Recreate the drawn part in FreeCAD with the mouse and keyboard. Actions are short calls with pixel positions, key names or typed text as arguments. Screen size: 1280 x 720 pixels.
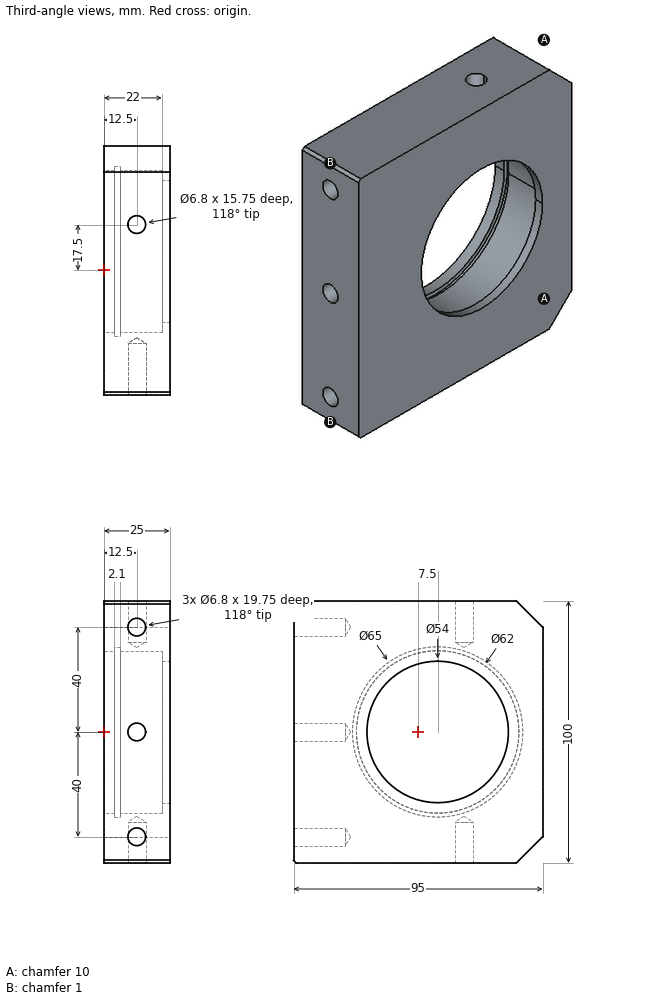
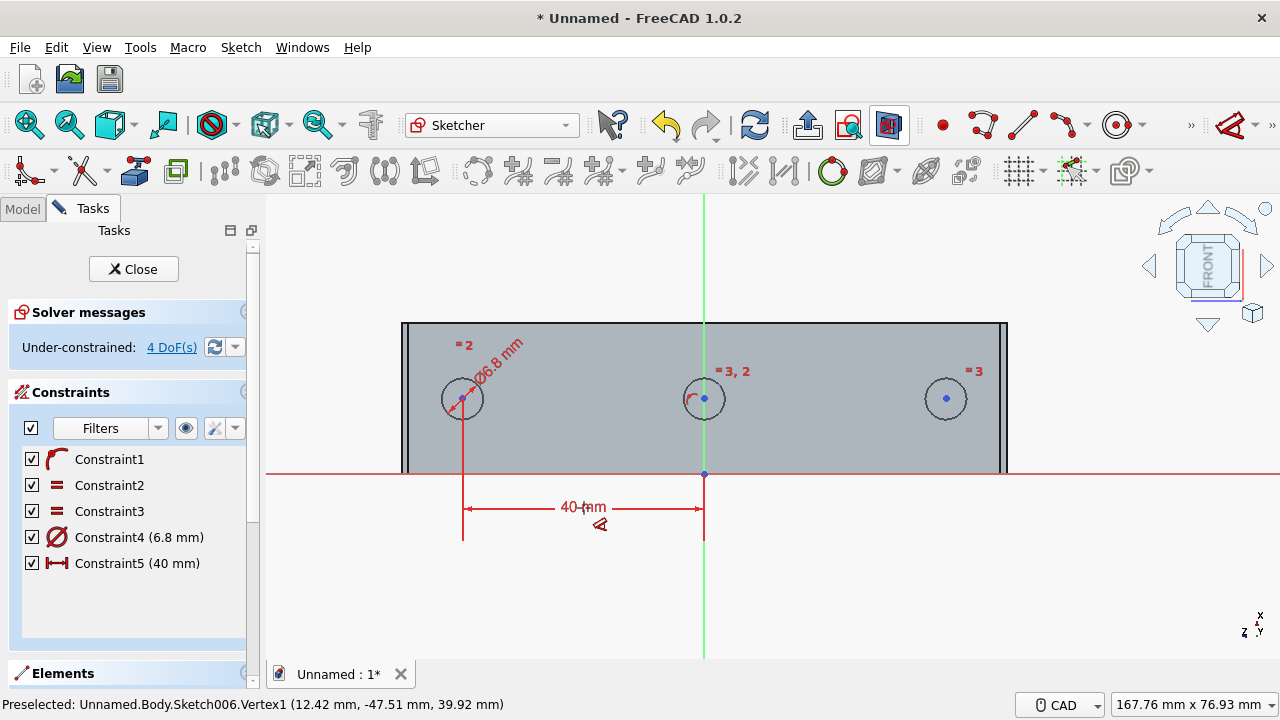
click(946, 399)
click(825, 508)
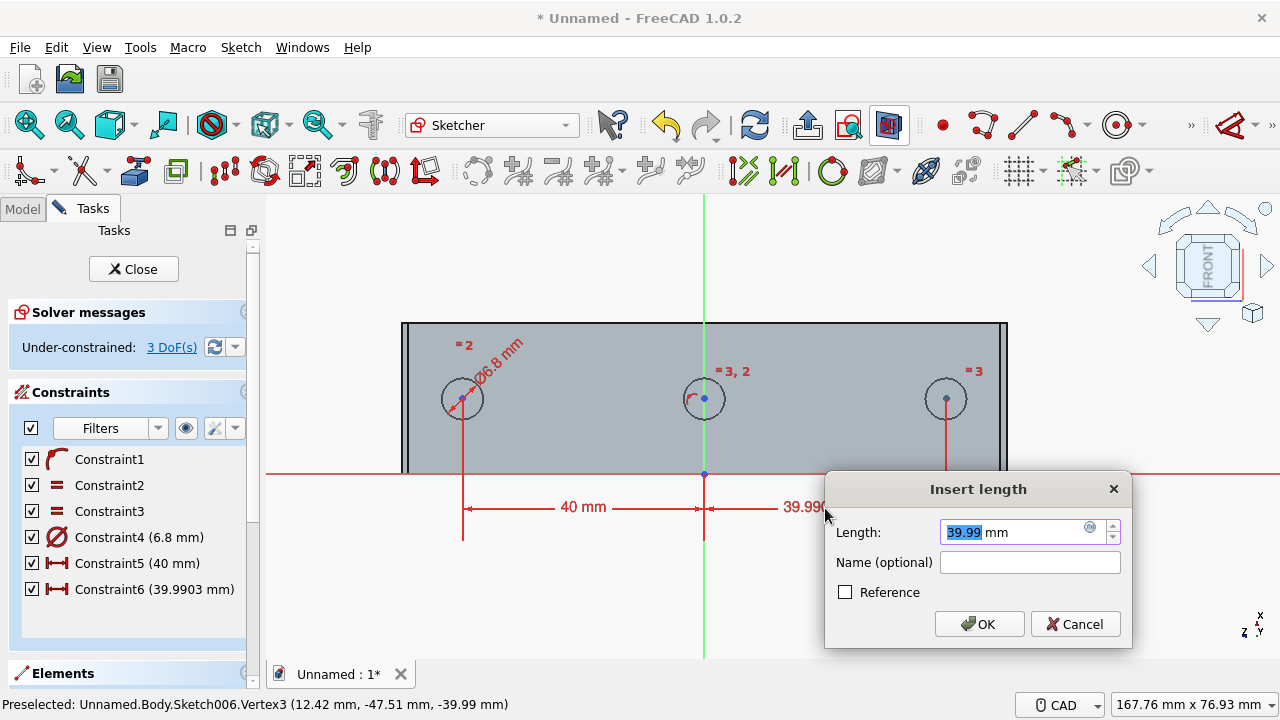
text(40)
key(Return)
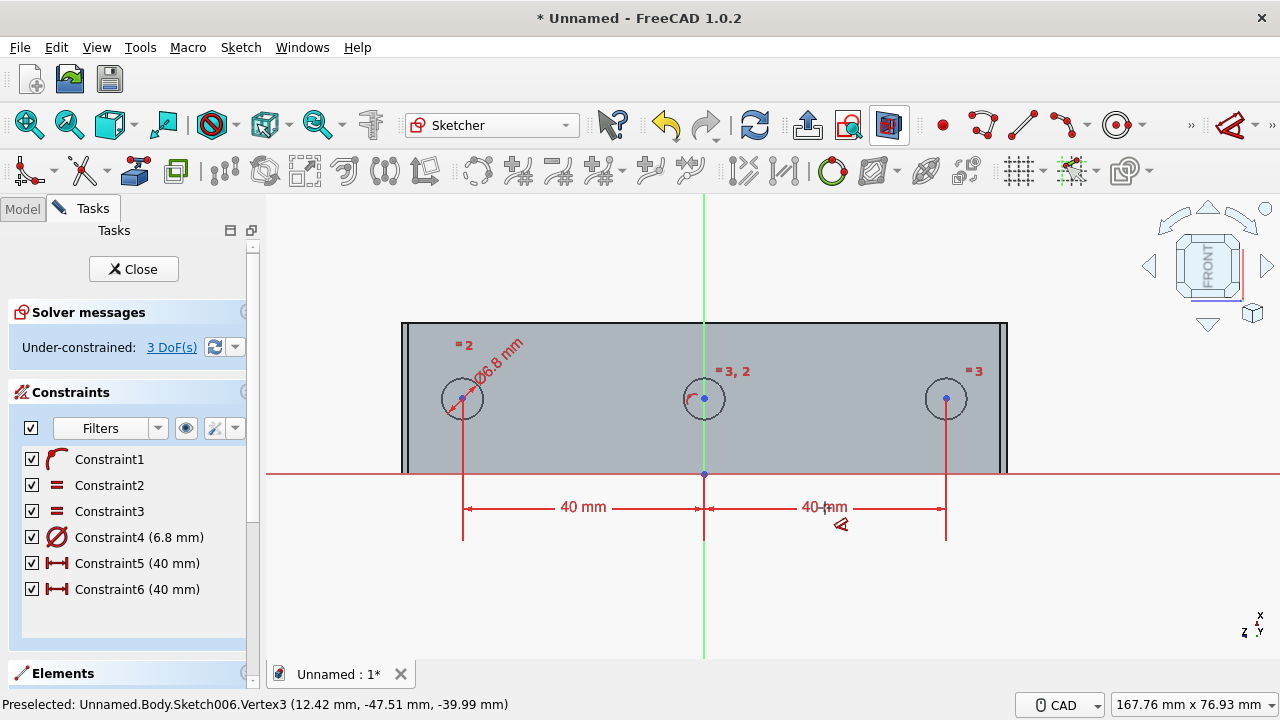
click(463, 399)
click(429, 437)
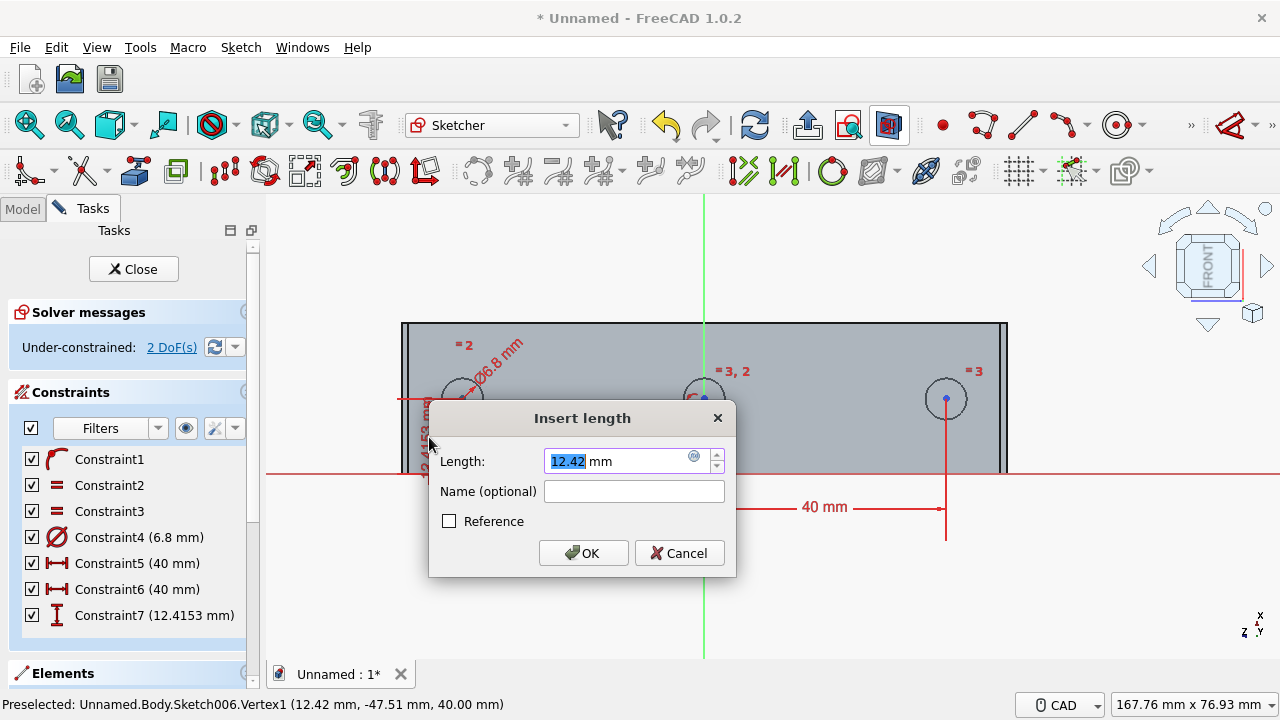
text(12.5)
key(Return)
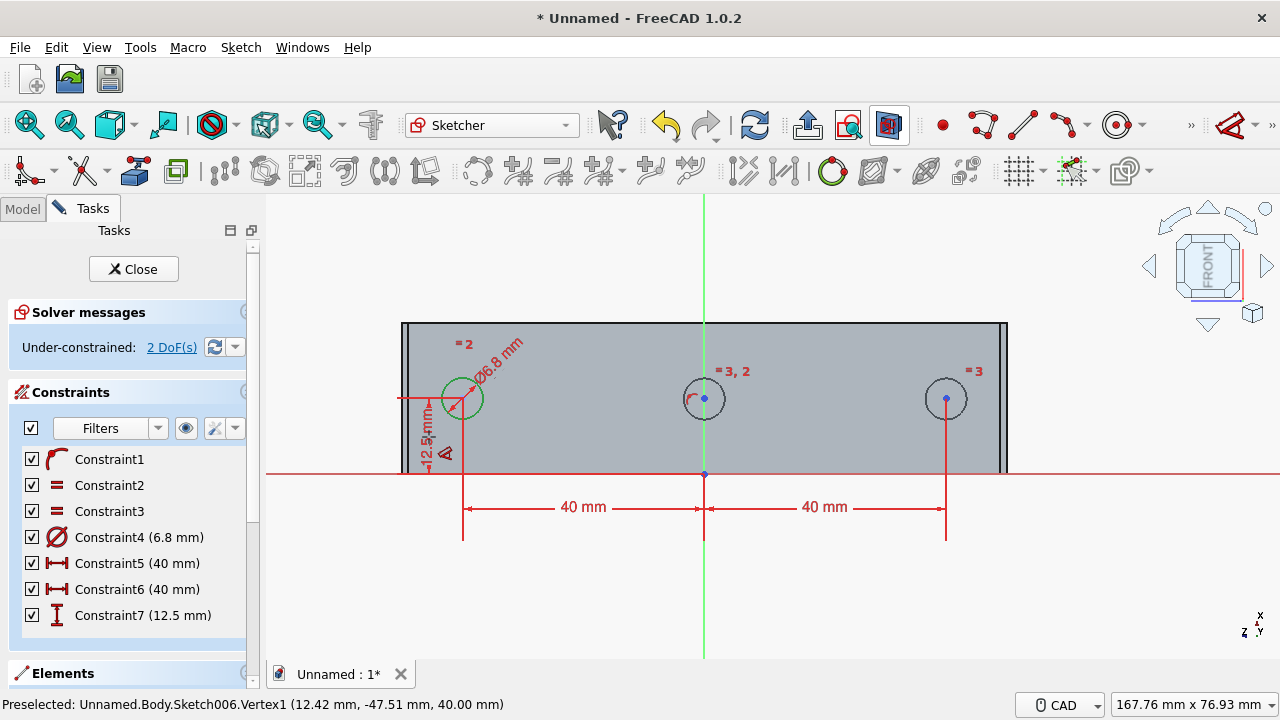
click(704, 399)
click(738, 437)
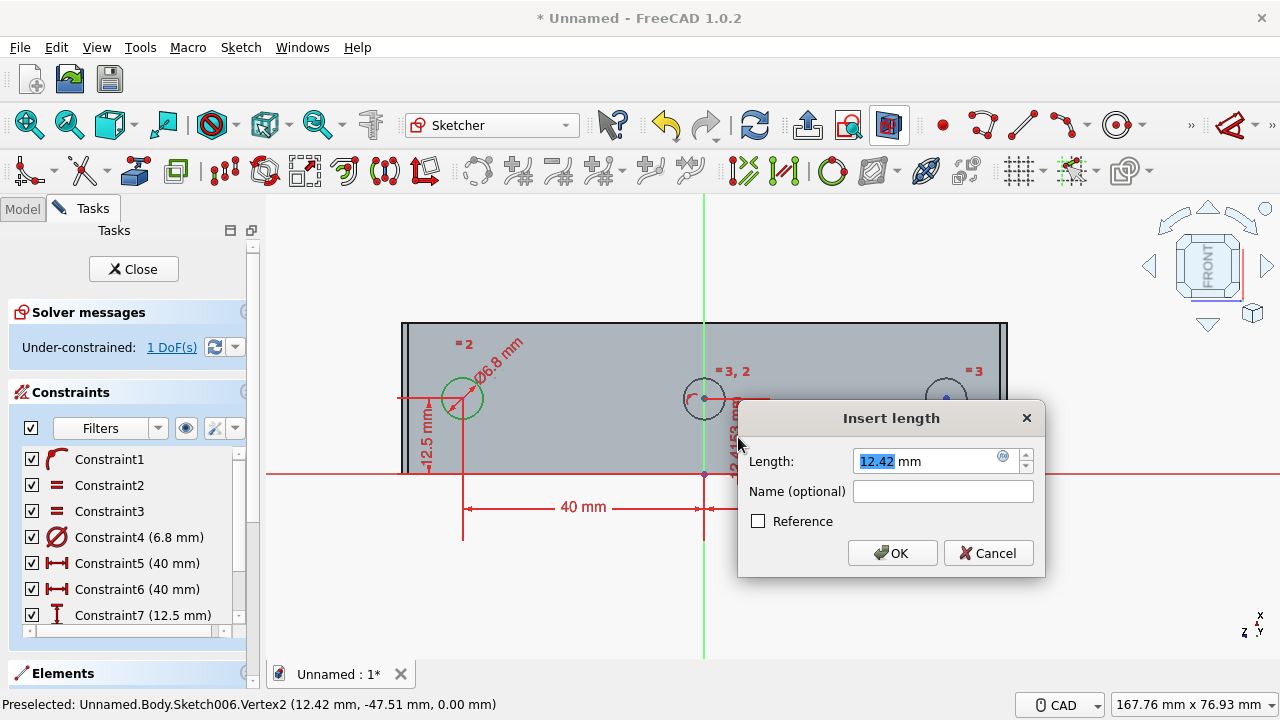
text(12.5)
key(Return)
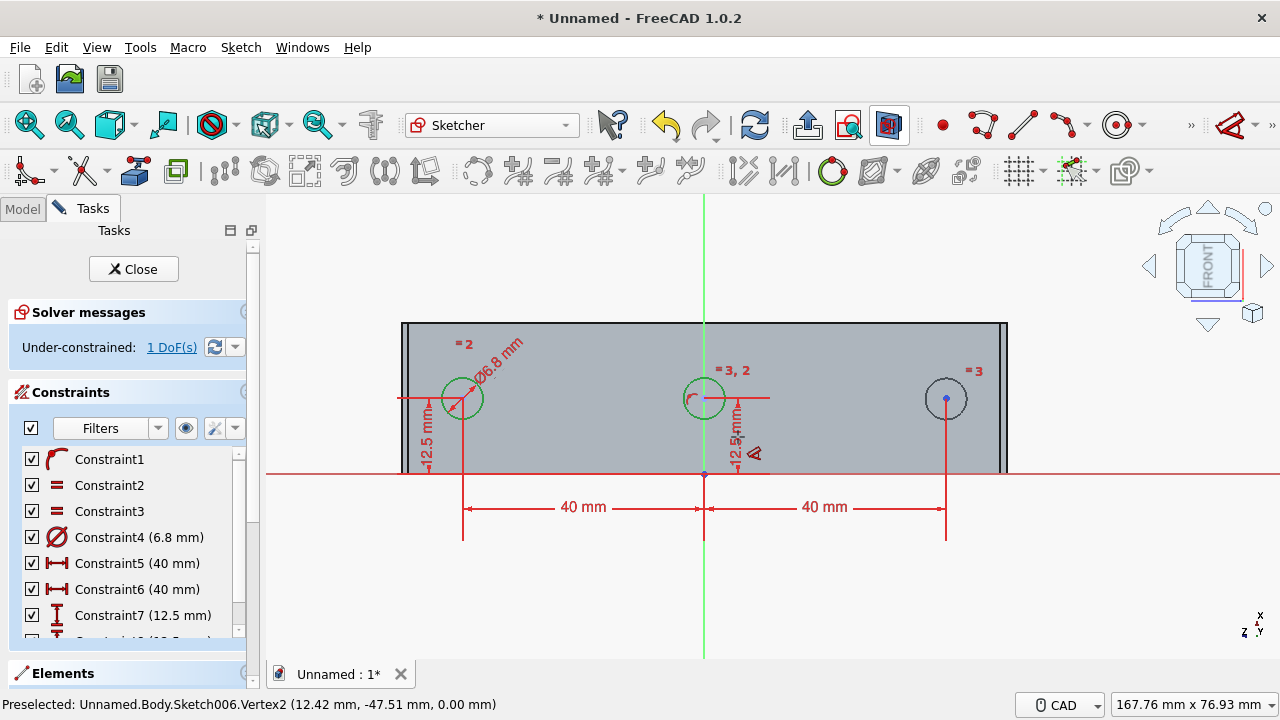
click(946, 399)
click(980, 437)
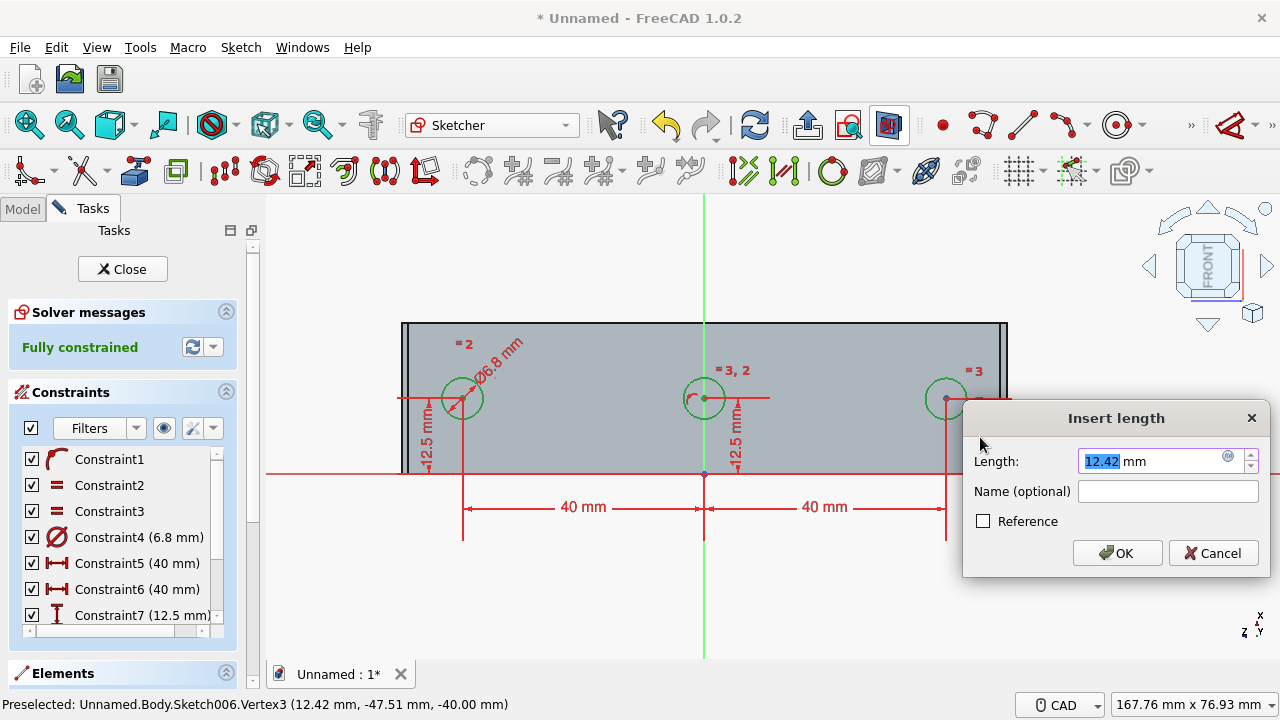
text(12.5)
key(Return)
key(Escape)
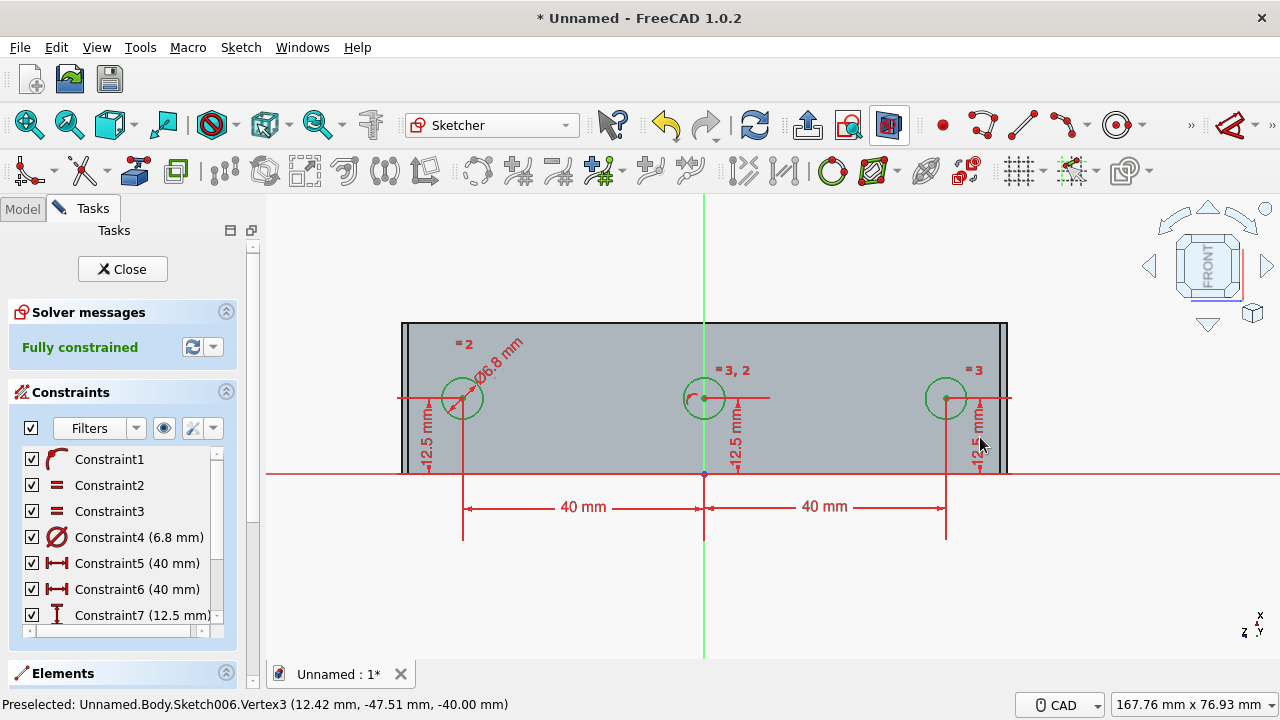
click(123, 269)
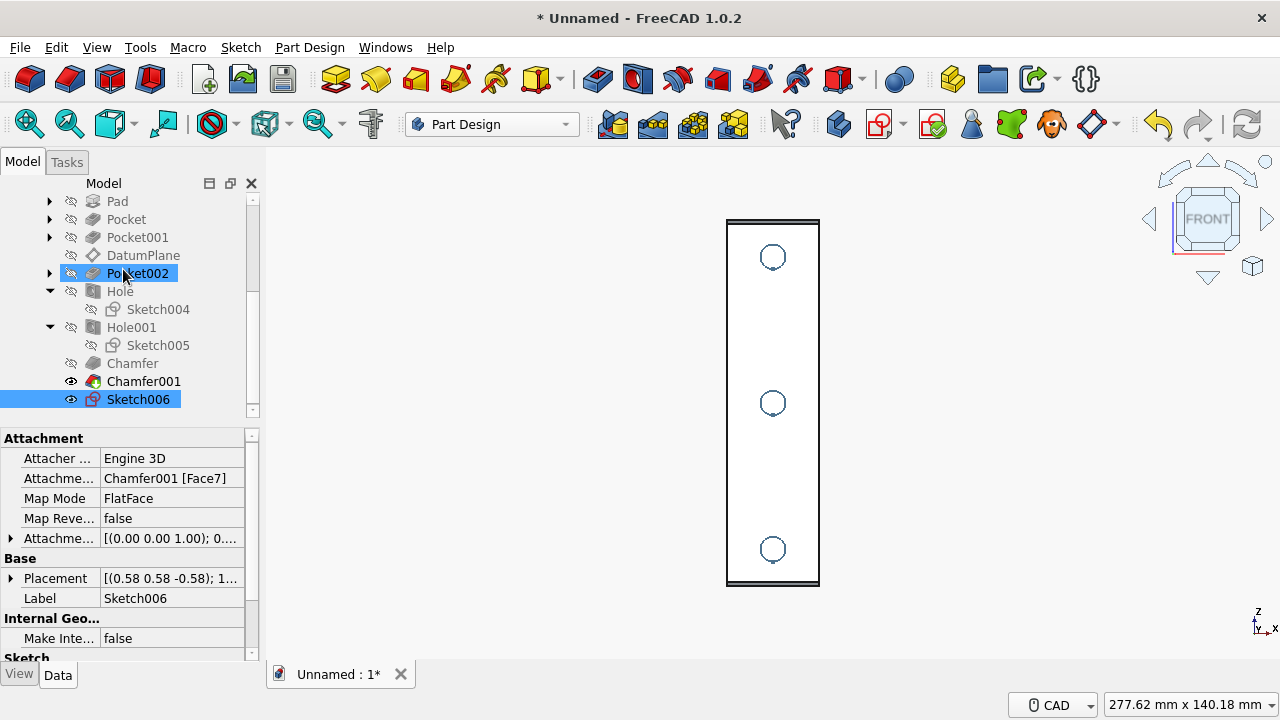
click(638, 80)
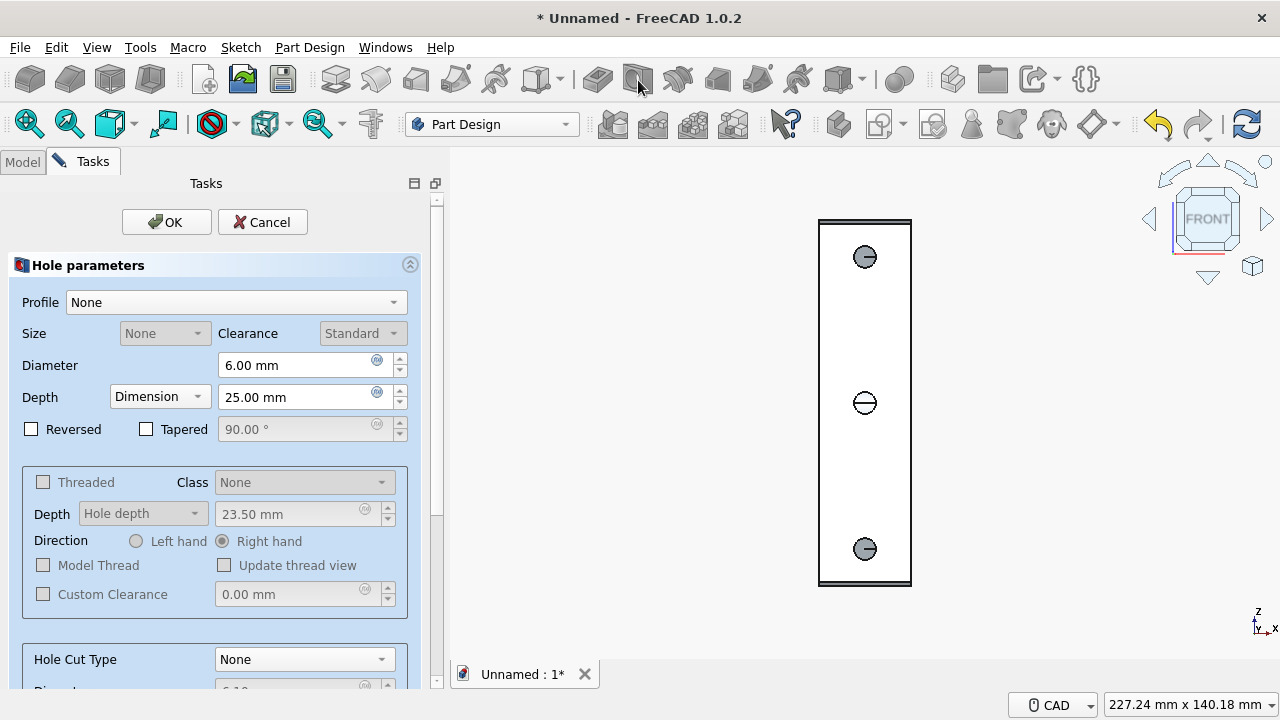
triple_click(305, 365)